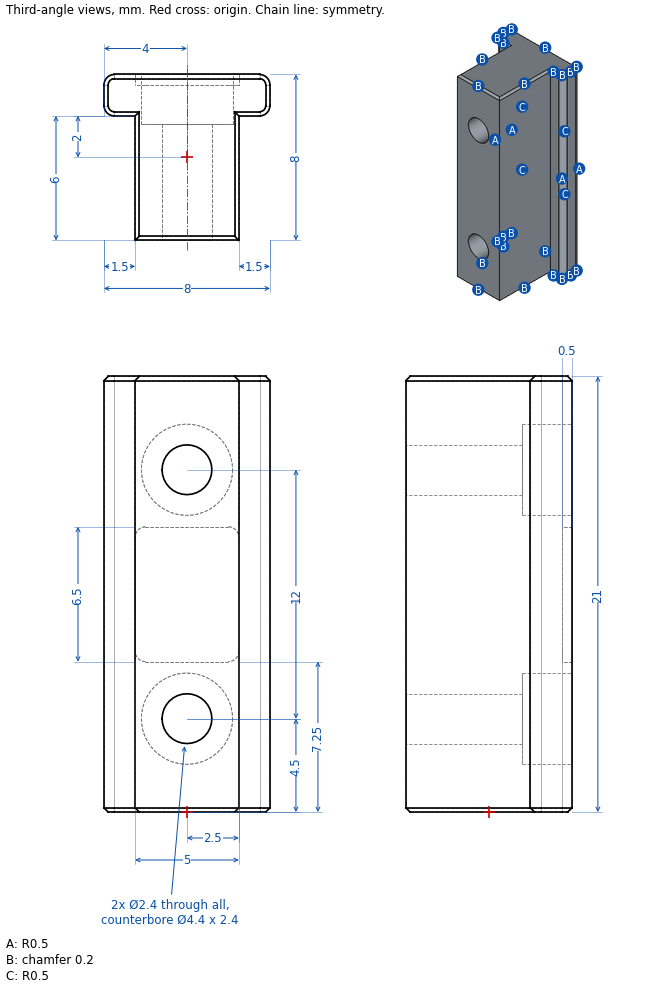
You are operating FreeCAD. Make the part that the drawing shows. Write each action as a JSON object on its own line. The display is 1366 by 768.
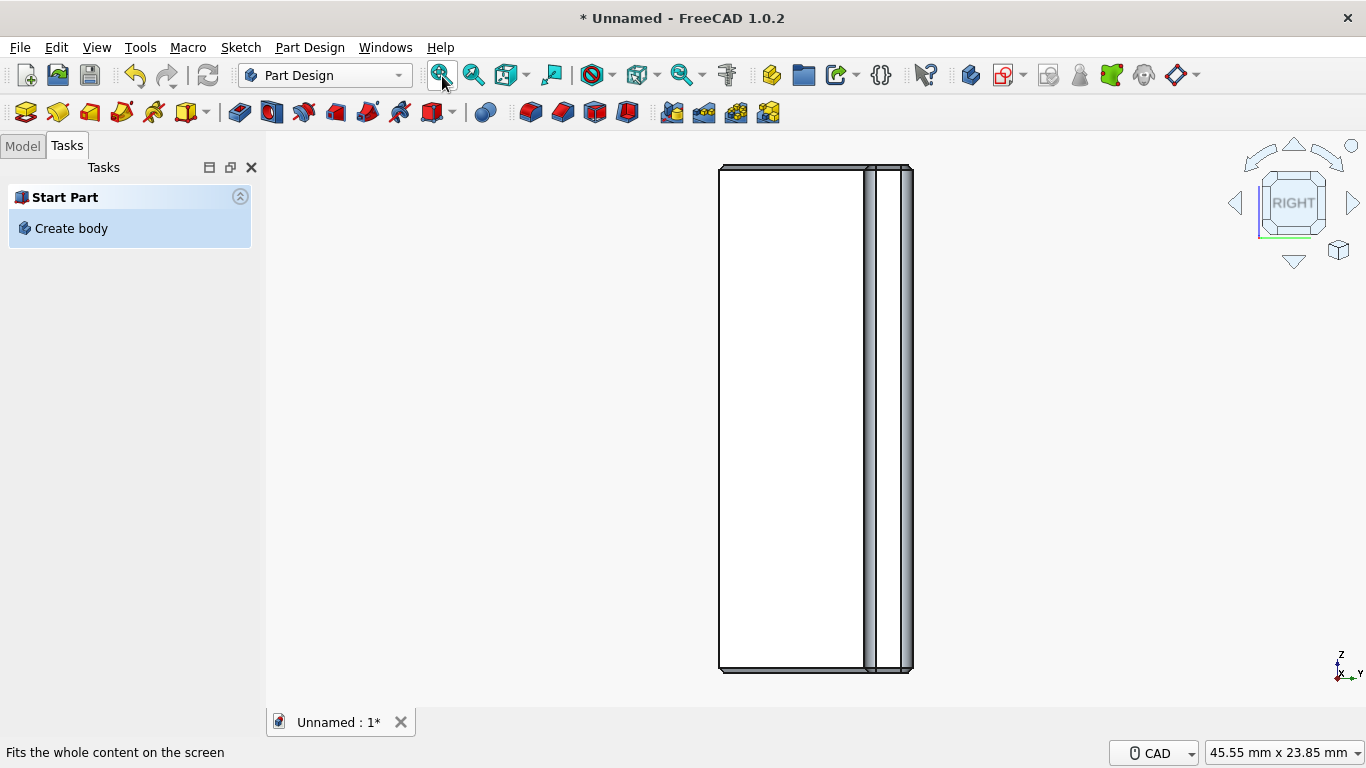
{"action": "key", "text": "5"}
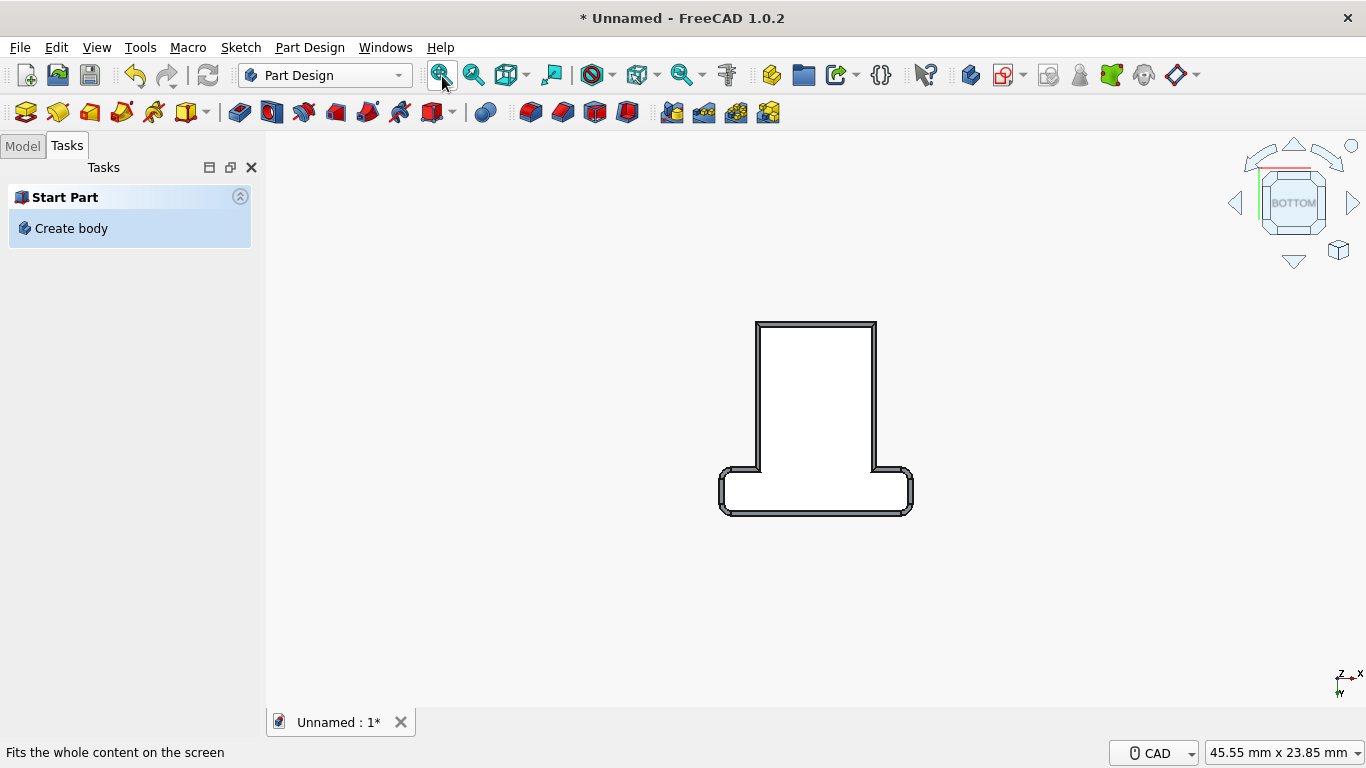
{"action": "left_click", "coordinate": [442, 76]}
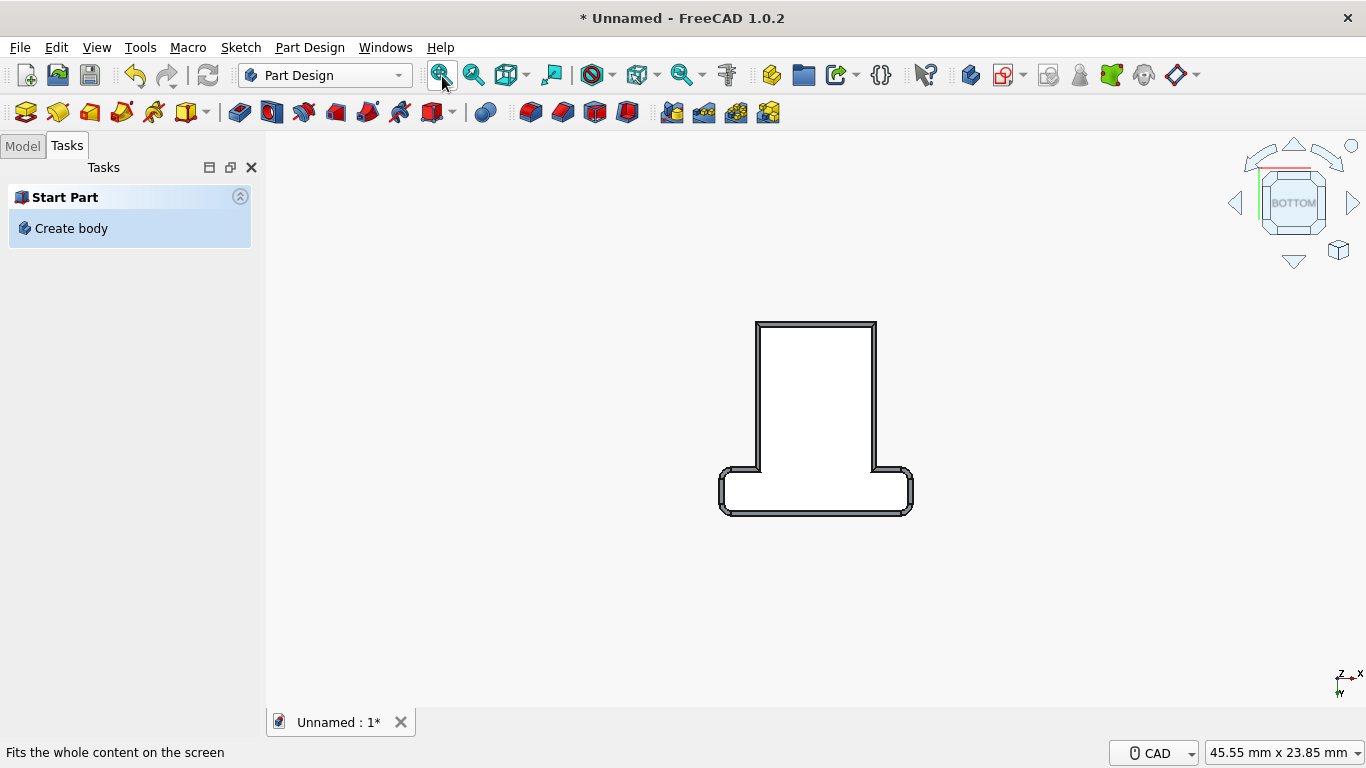
{"action": "scroll", "coordinate": [876, 509], "scroll_direction": "up", "scroll_amount": 6}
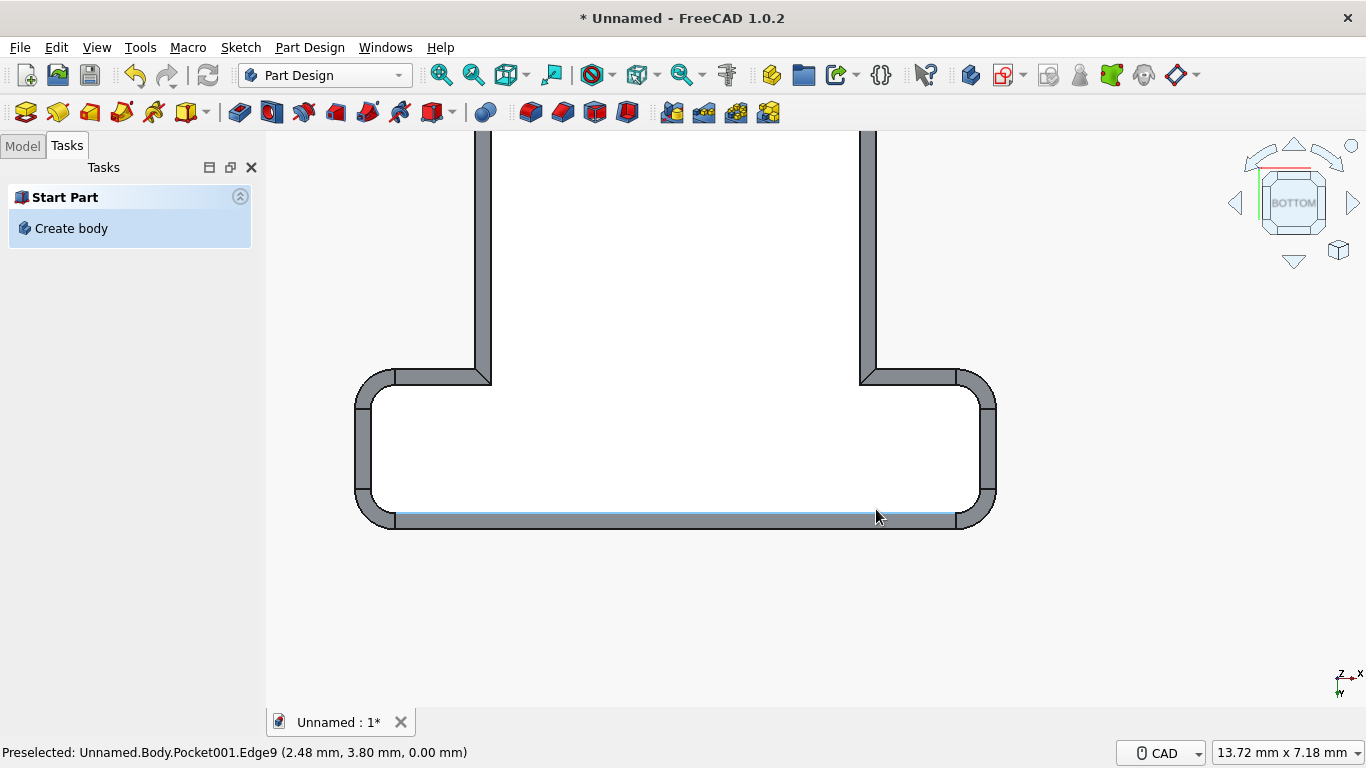
{"action": "left_click", "coordinate": [442, 76]}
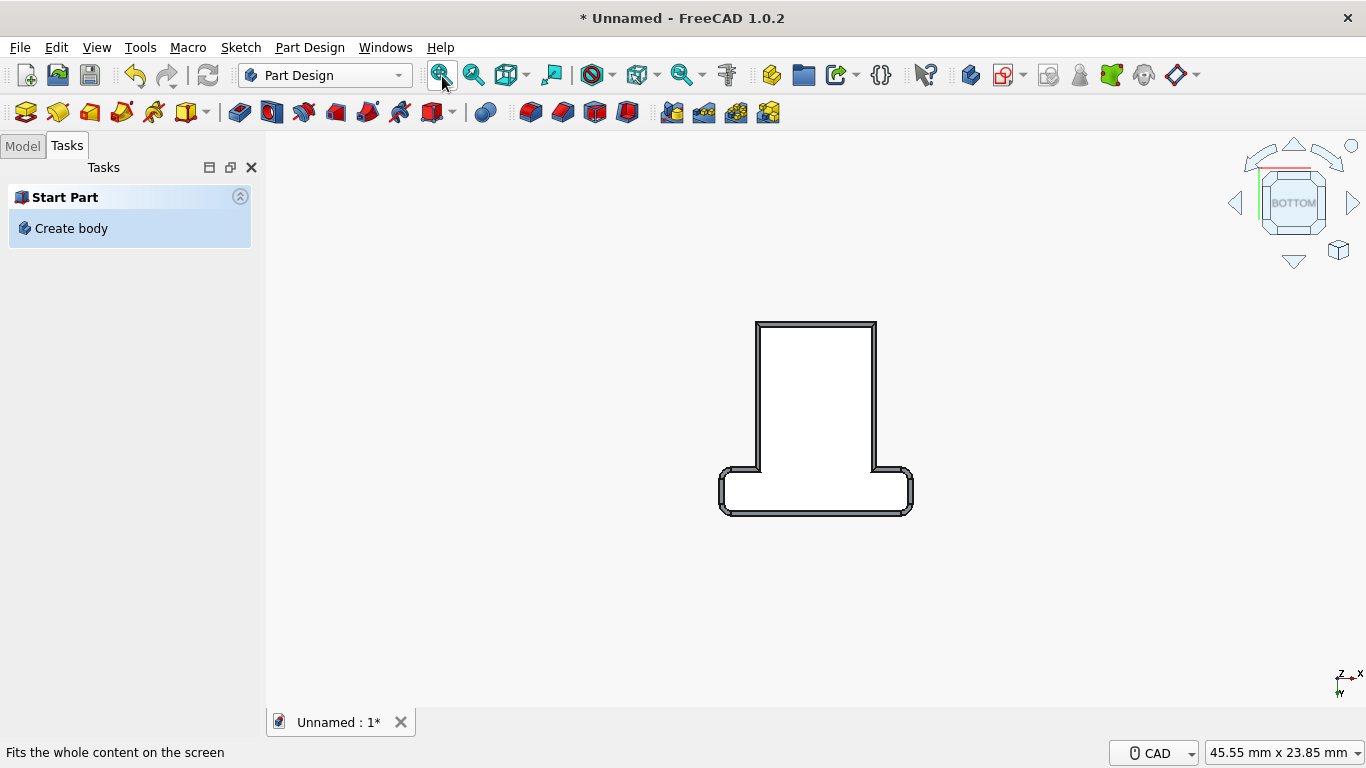
{"action": "key", "text": "4"}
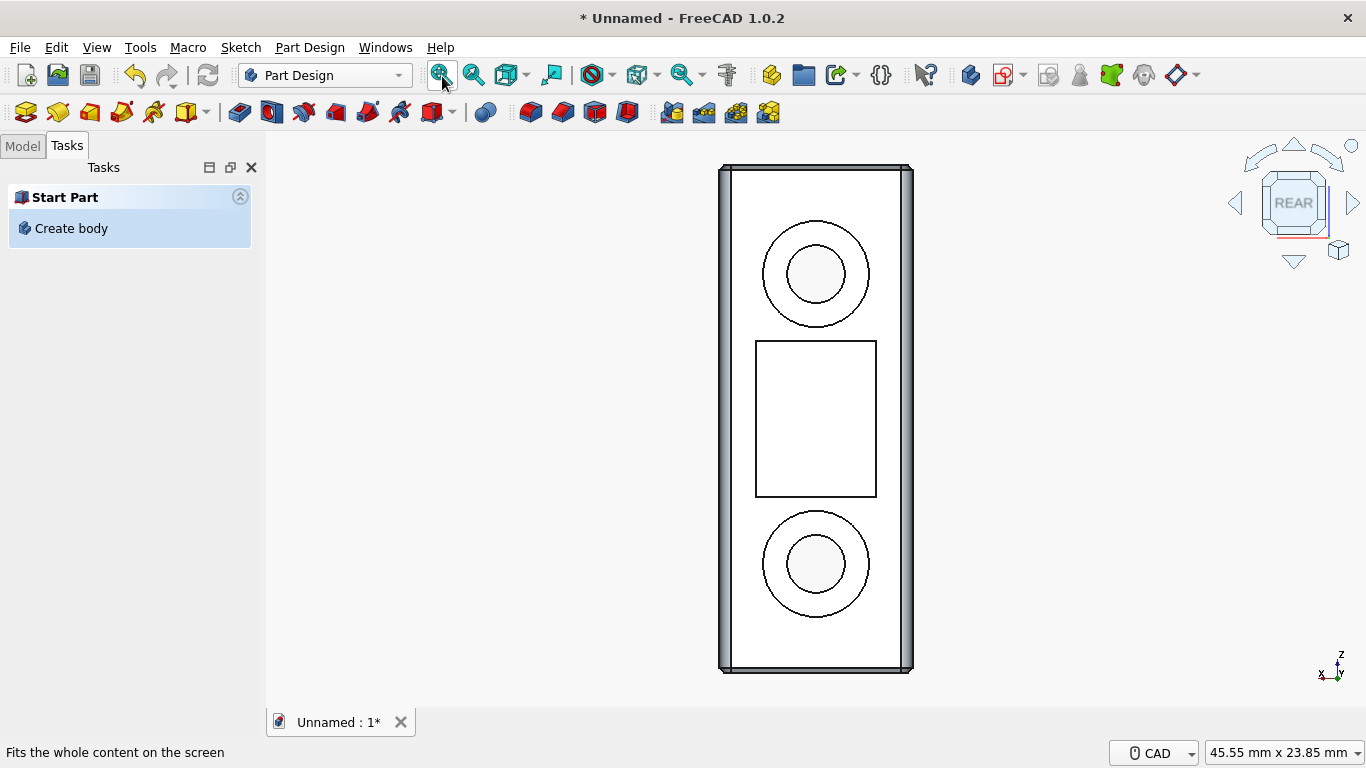
{"action": "scroll", "coordinate": [756, 496], "scroll_direction": "up", "scroll_amount": 6}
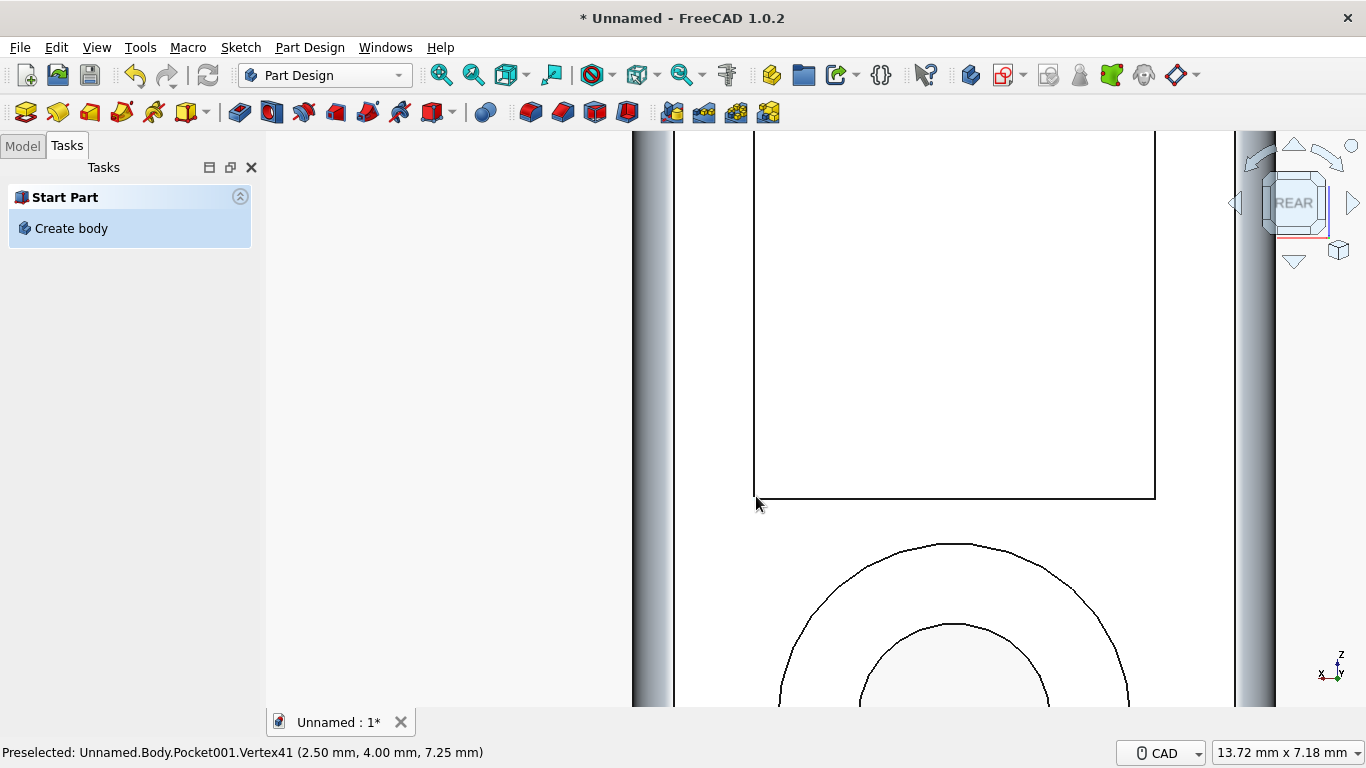
{"action": "left_click", "coordinate": [442, 76]}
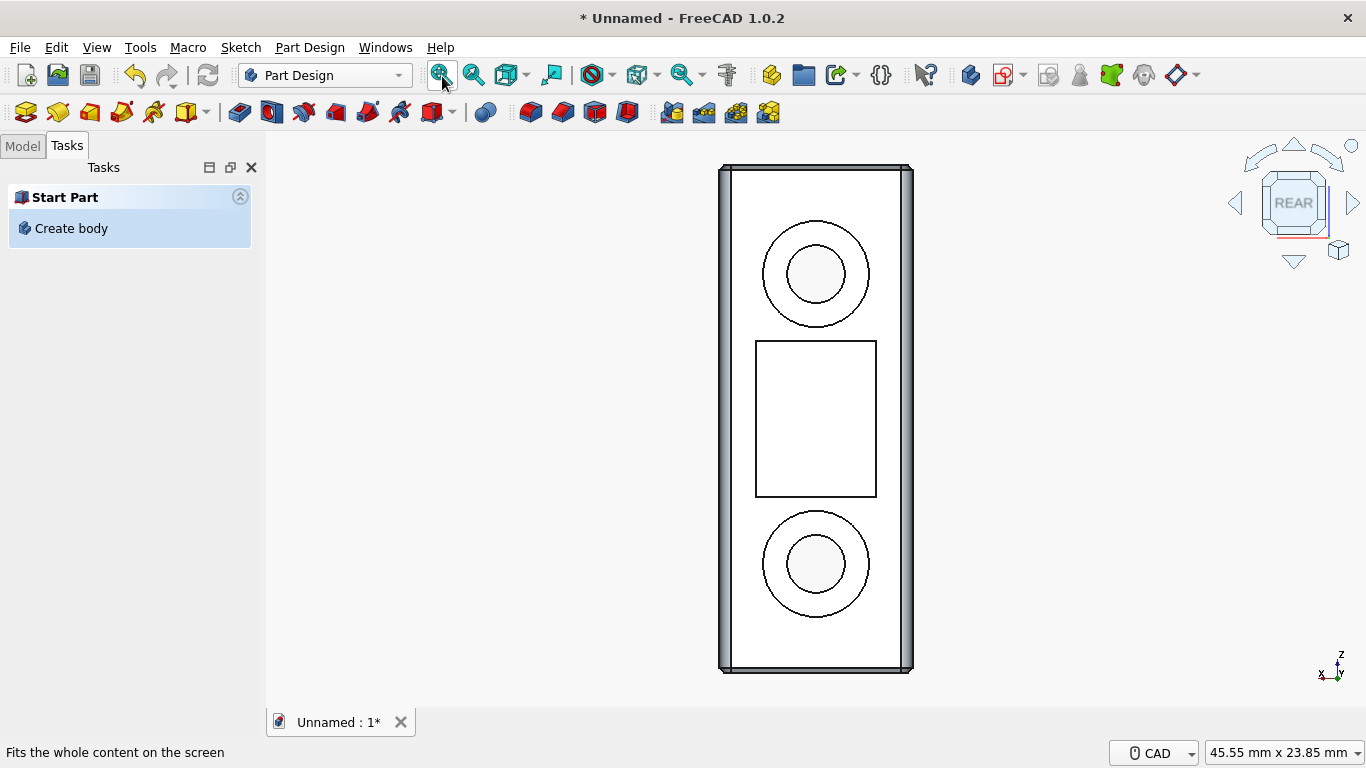
{"action": "key", "text": "6"}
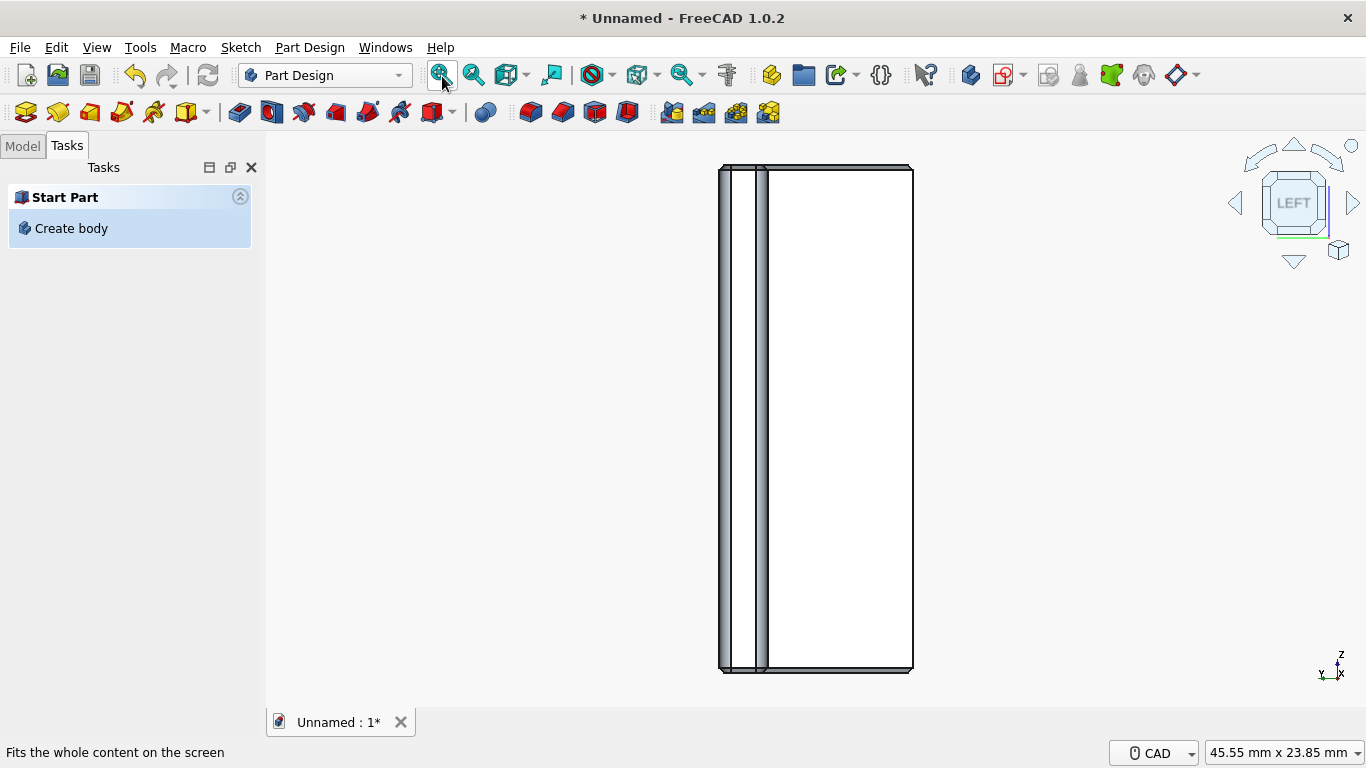
{"action": "scroll", "coordinate": [725, 496], "scroll_direction": "up", "scroll_amount": 6}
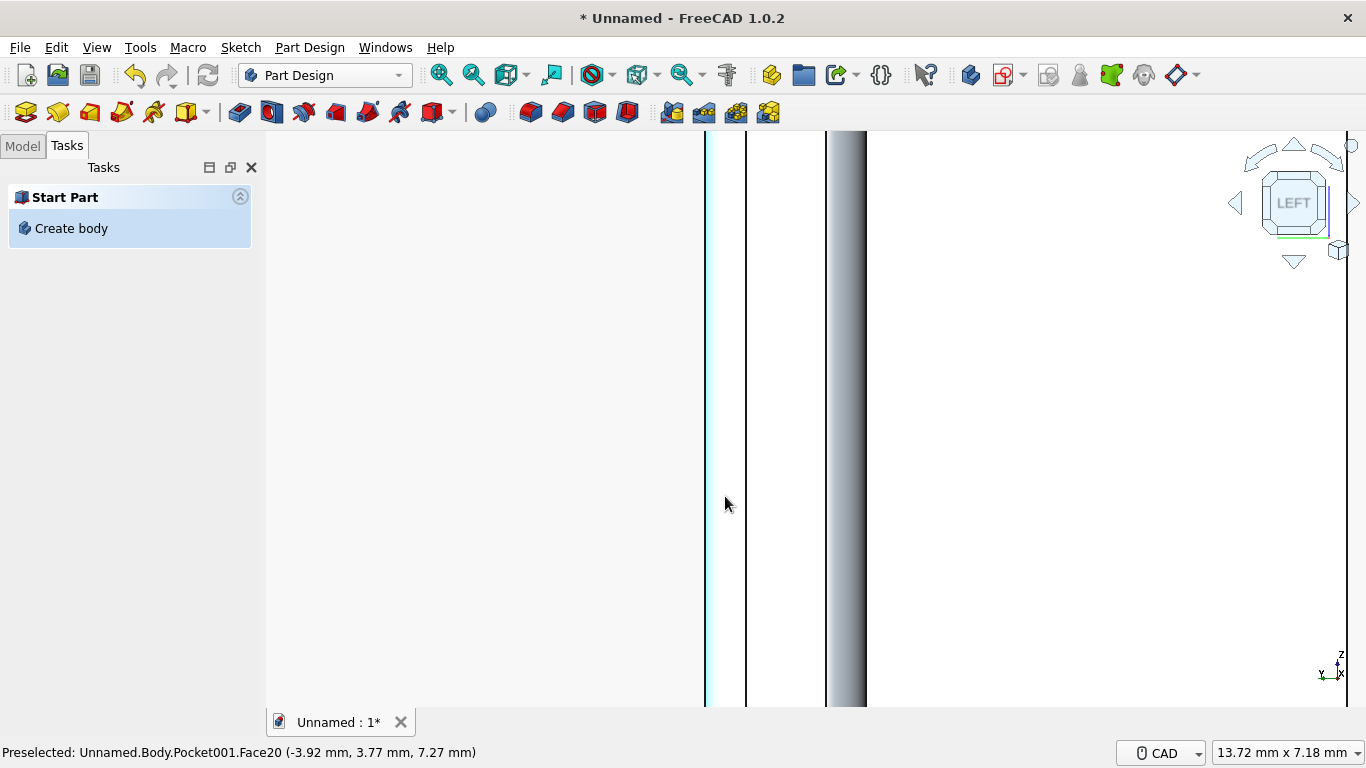
{"action": "left_click", "coordinate": [442, 76]}